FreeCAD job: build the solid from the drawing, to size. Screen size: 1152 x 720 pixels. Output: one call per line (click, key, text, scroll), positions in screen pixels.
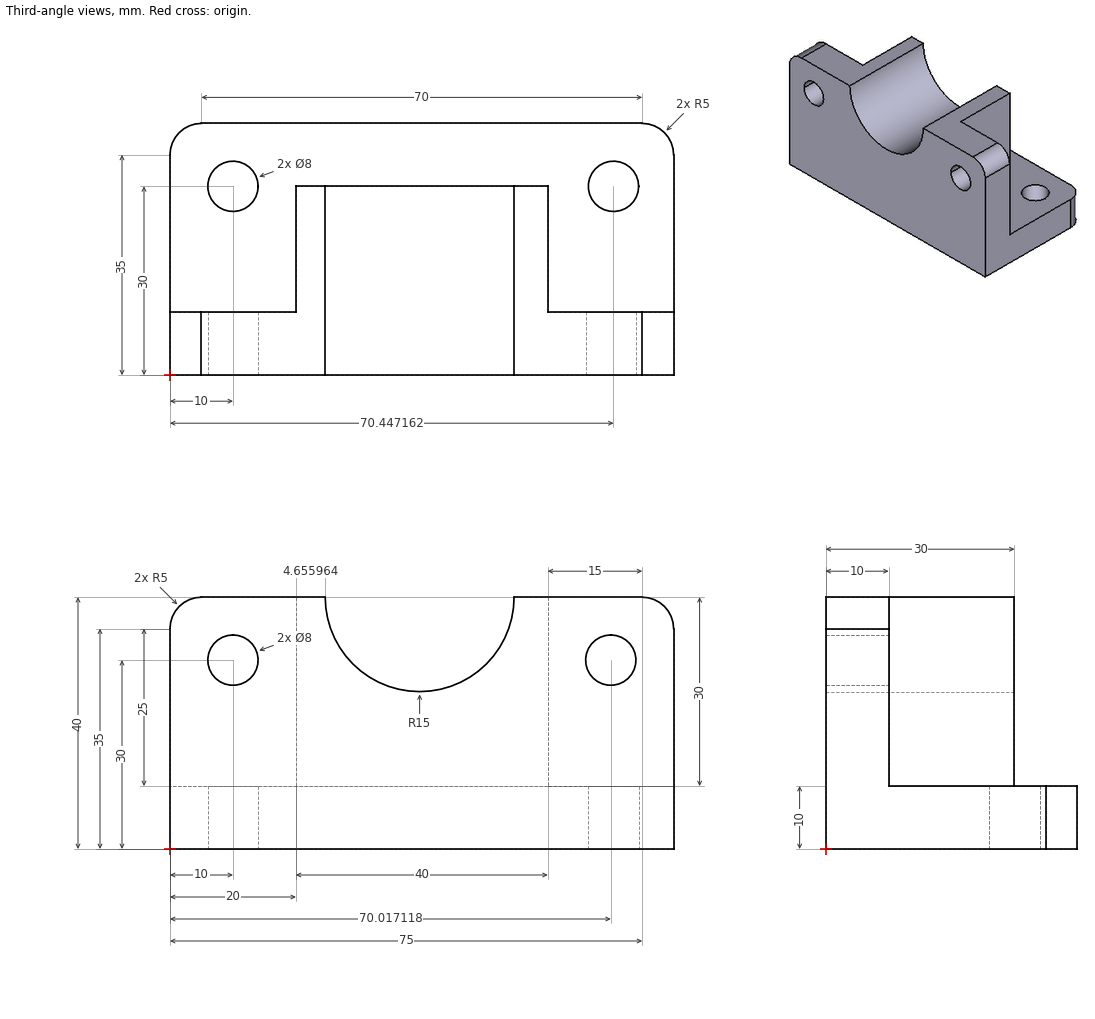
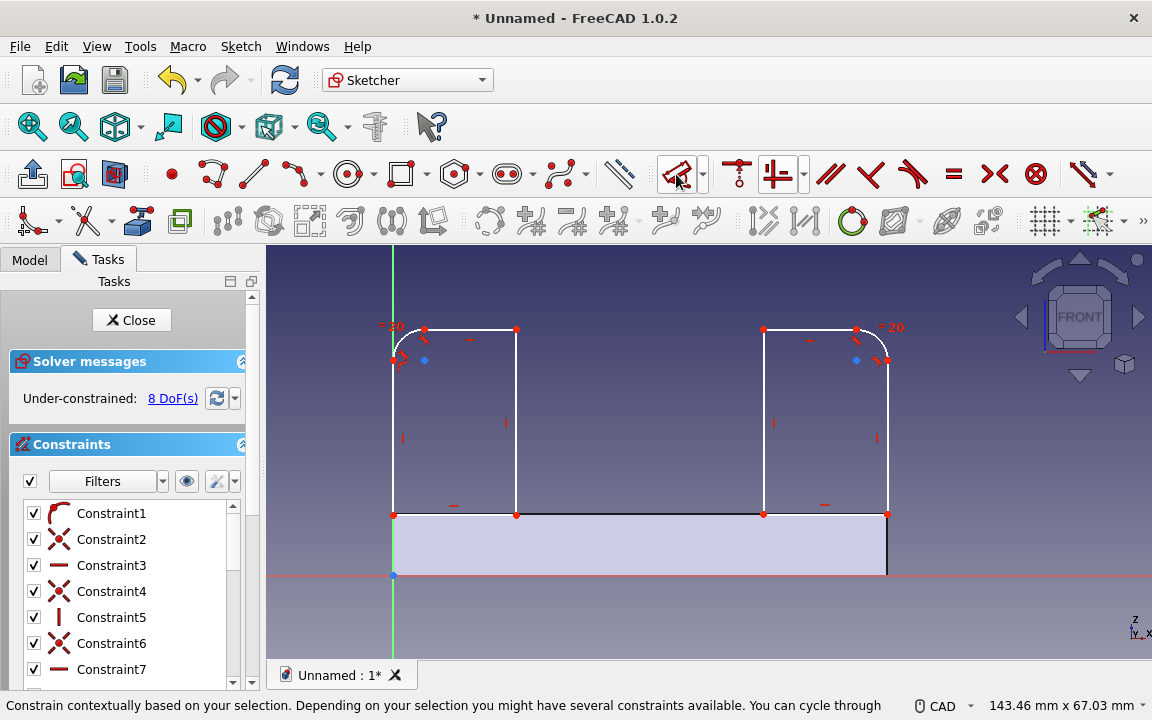
scroll(410, 333, up, 2)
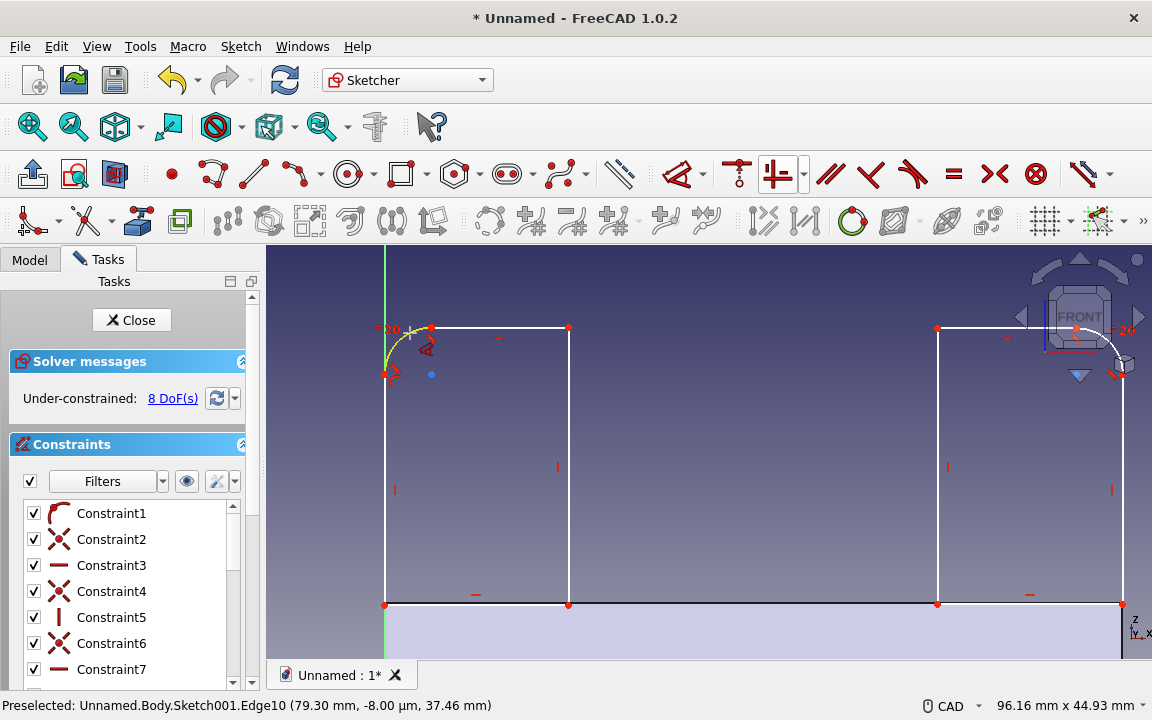
click(410, 333)
click(433, 296)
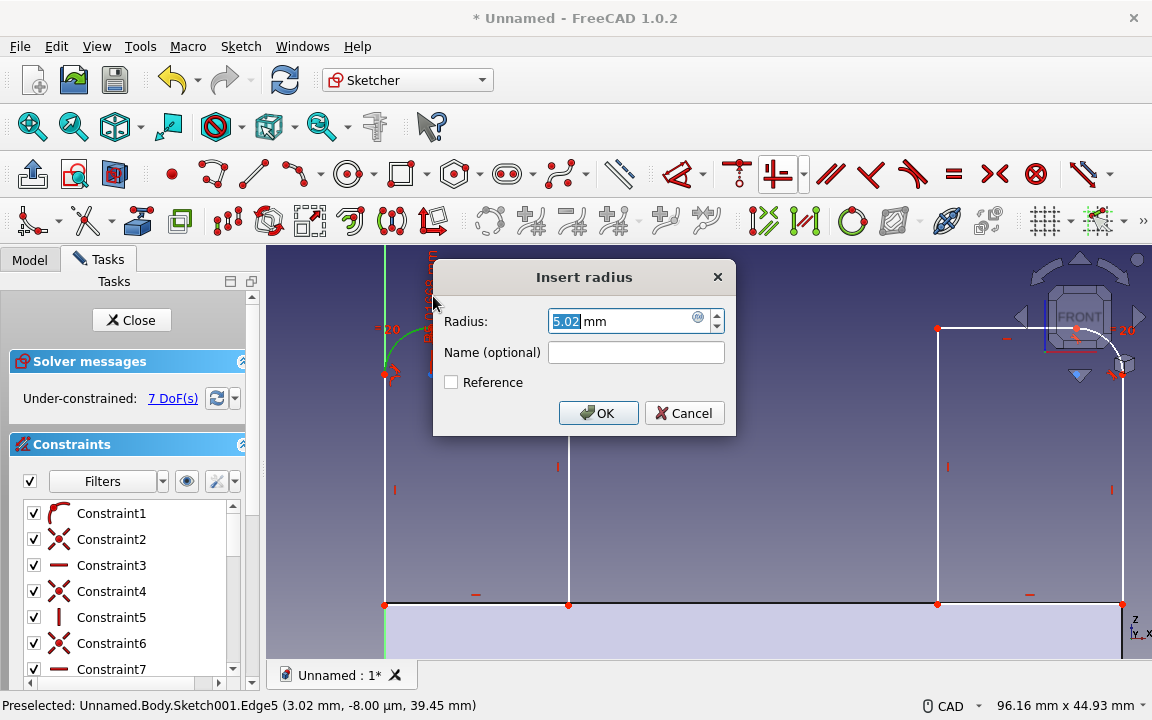
text(5)
key(Return)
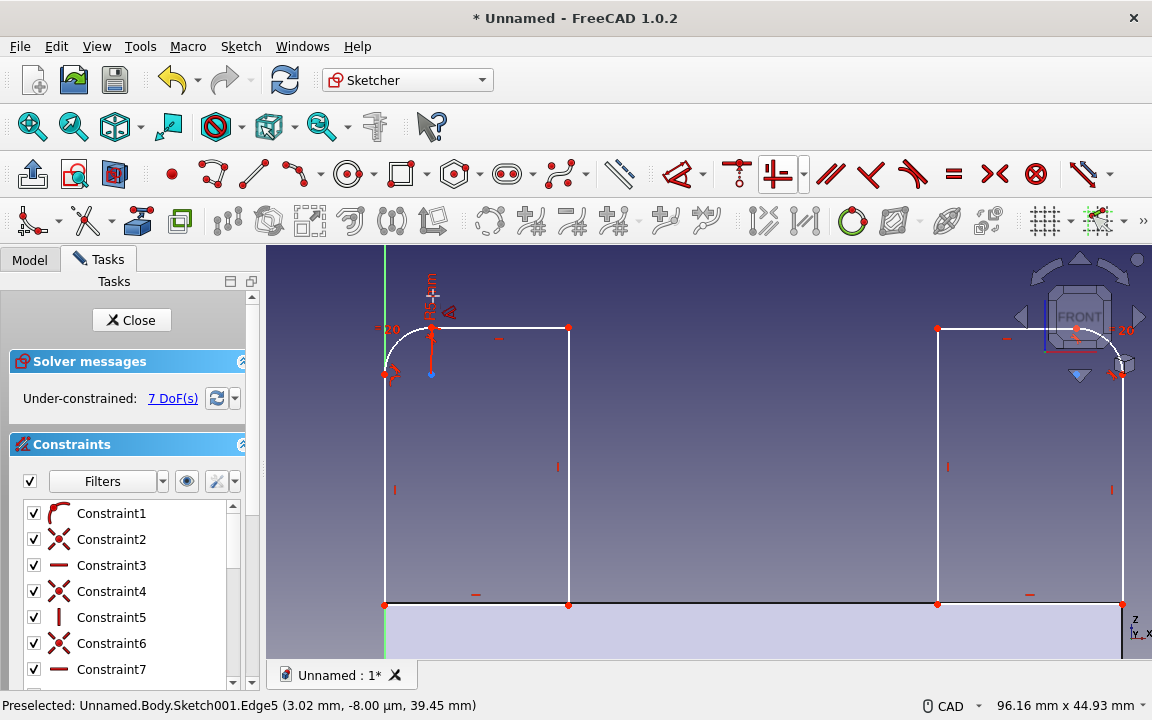
click(385, 443)
click(351, 490)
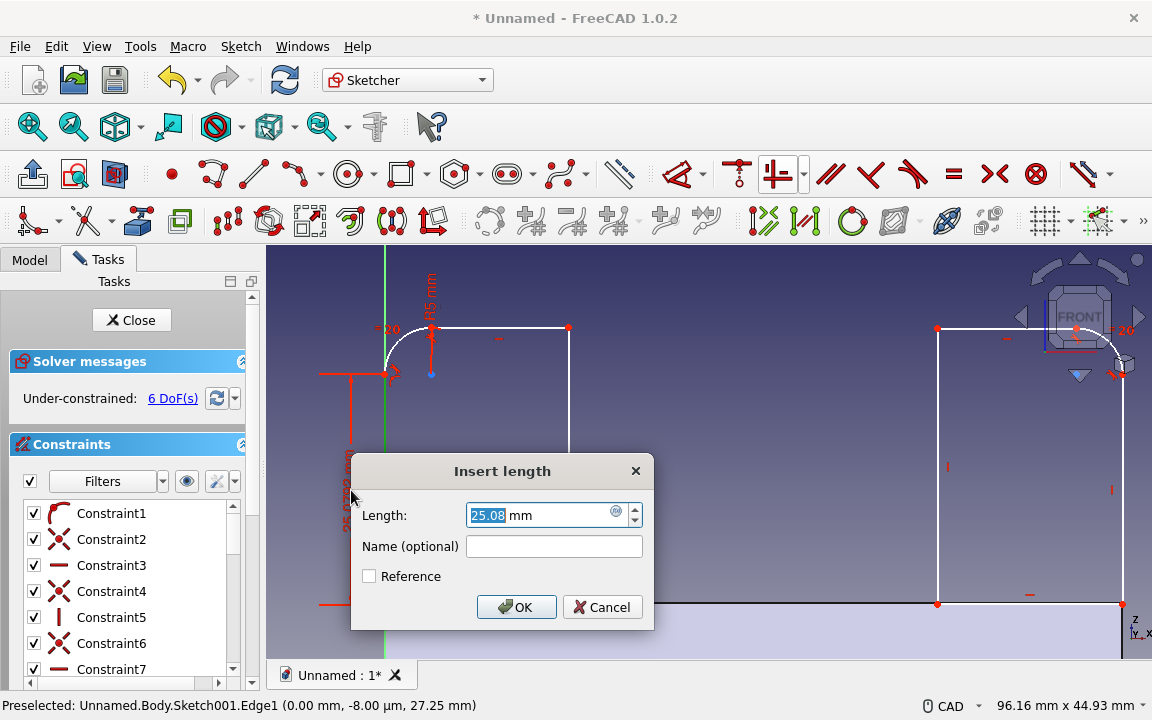
text(25)
key(Return)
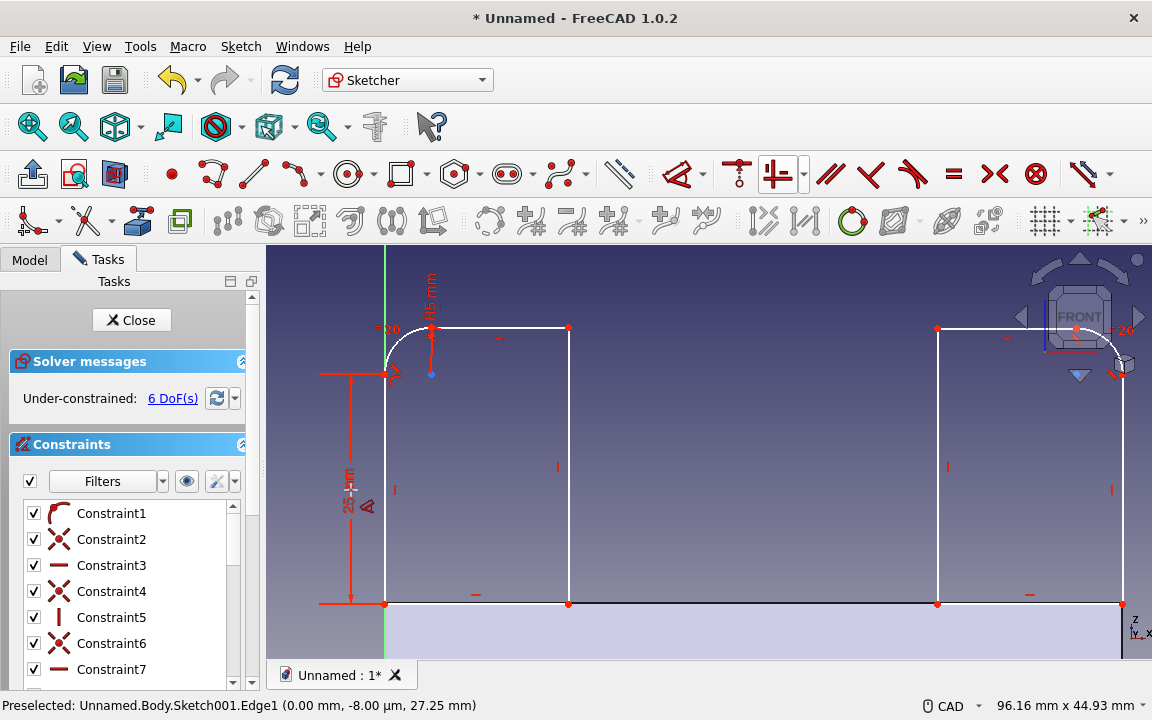
click(440, 604)
click(477, 570)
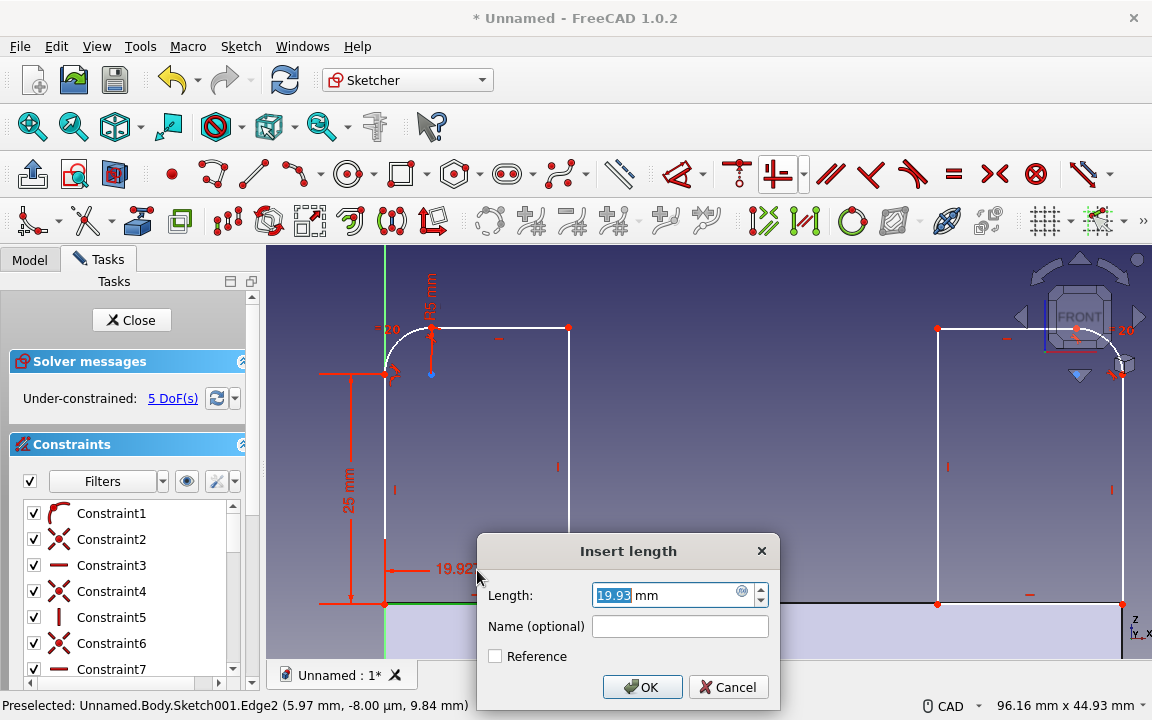
text(20)
key(Return)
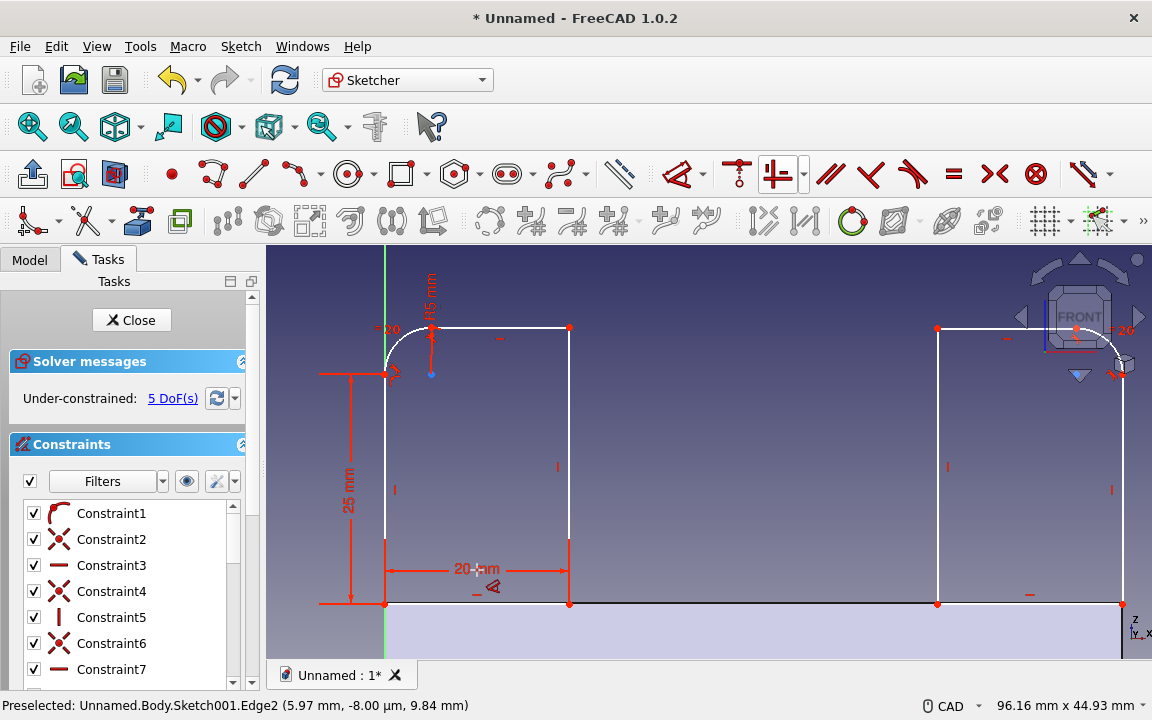
click(980, 329)
click(962, 295)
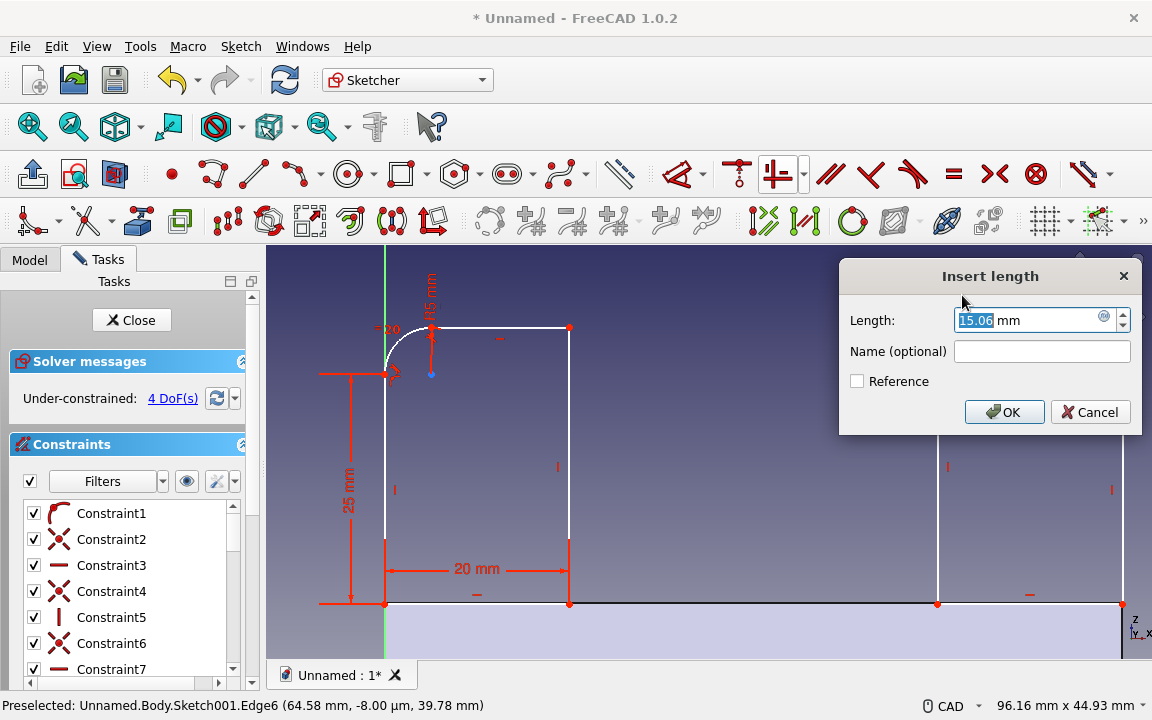
text(15)
key(Return)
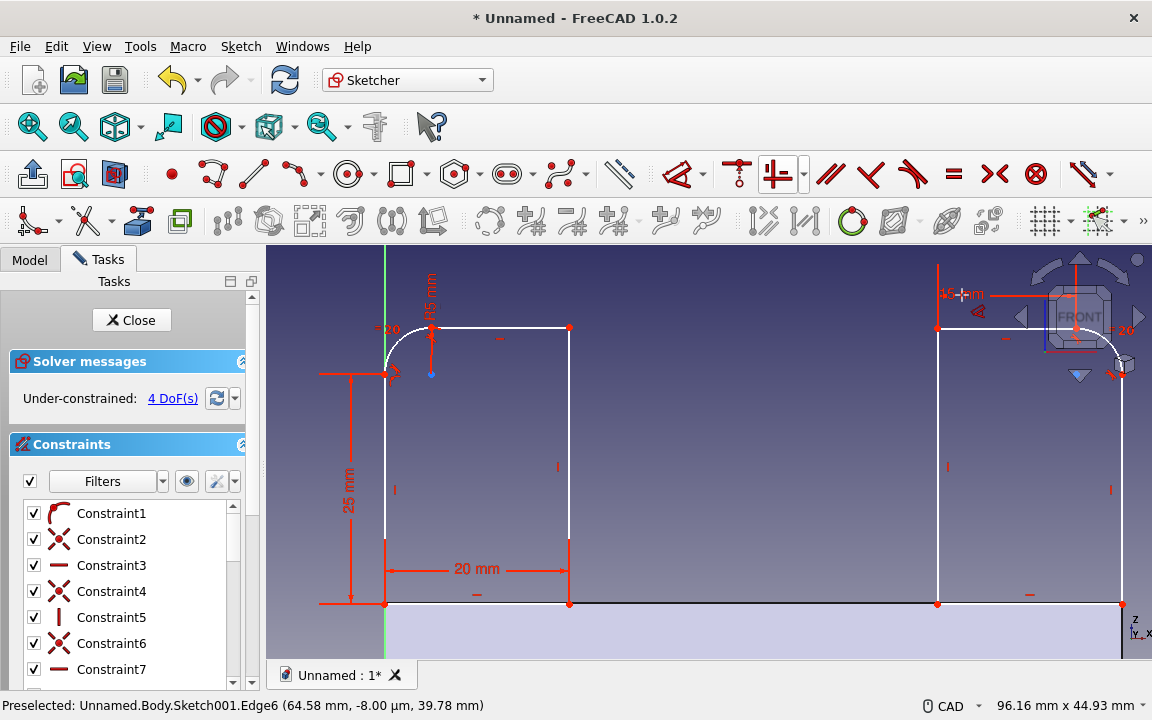
click(938, 411)
click(972, 466)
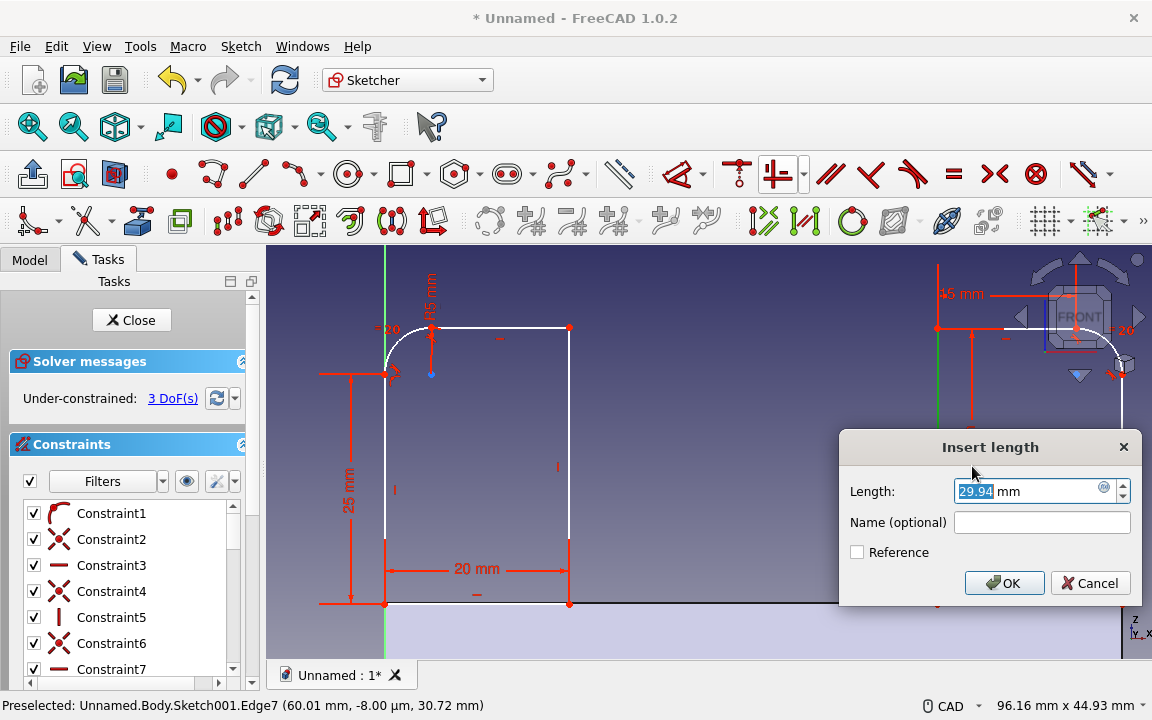
text(30)
key(Return)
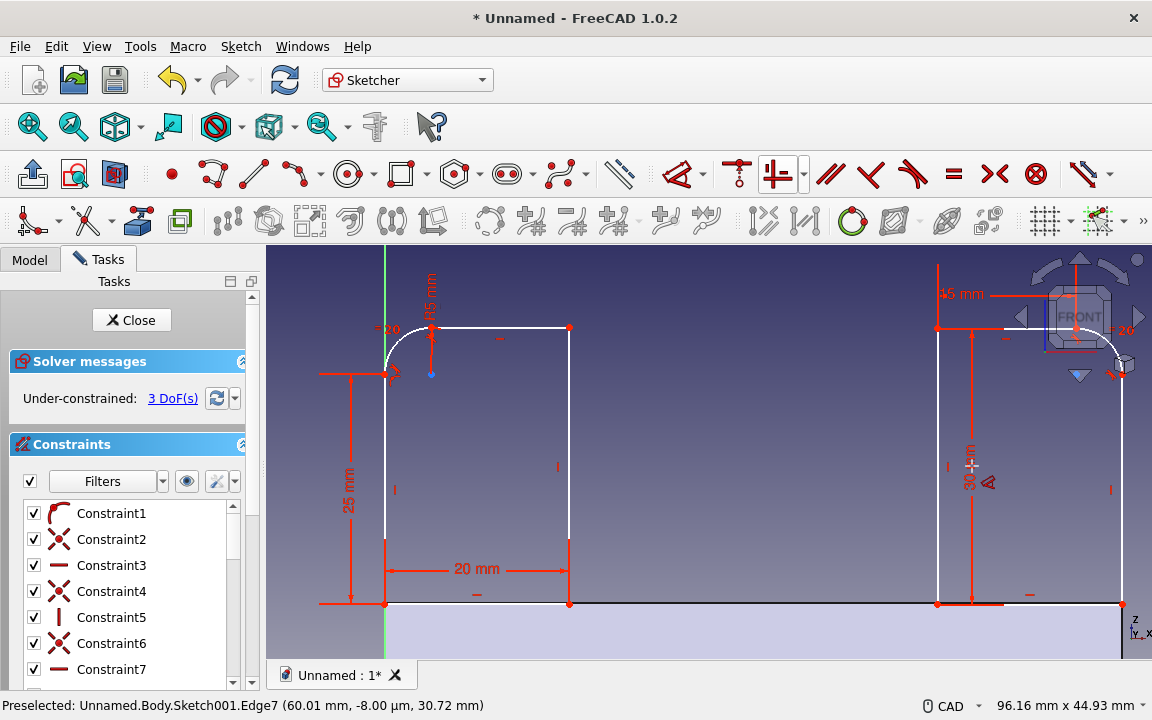
click(385, 374)
click(351, 443)